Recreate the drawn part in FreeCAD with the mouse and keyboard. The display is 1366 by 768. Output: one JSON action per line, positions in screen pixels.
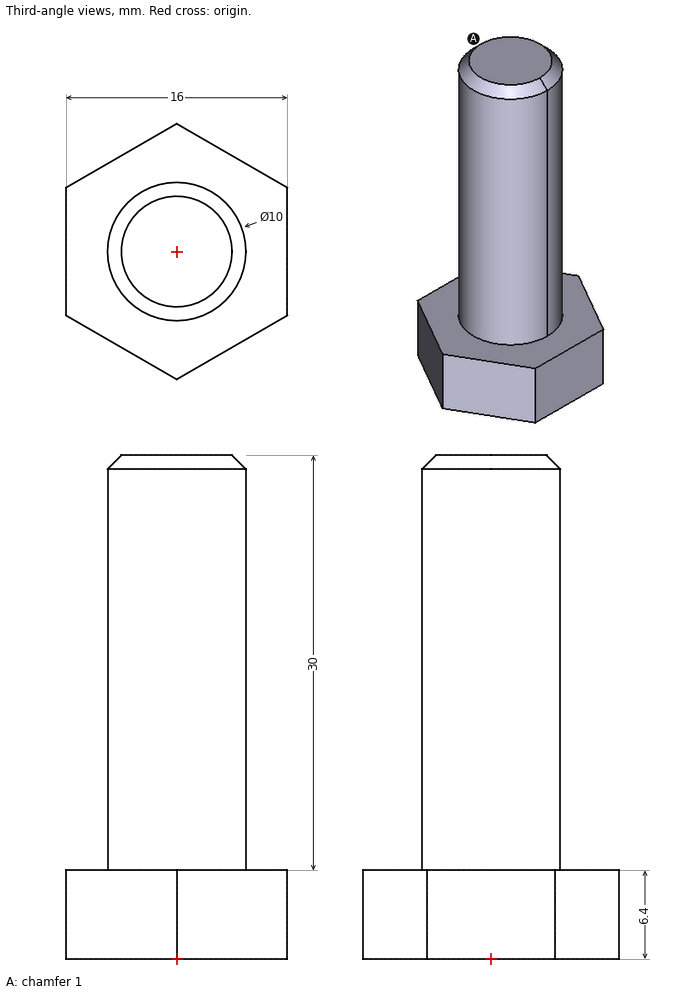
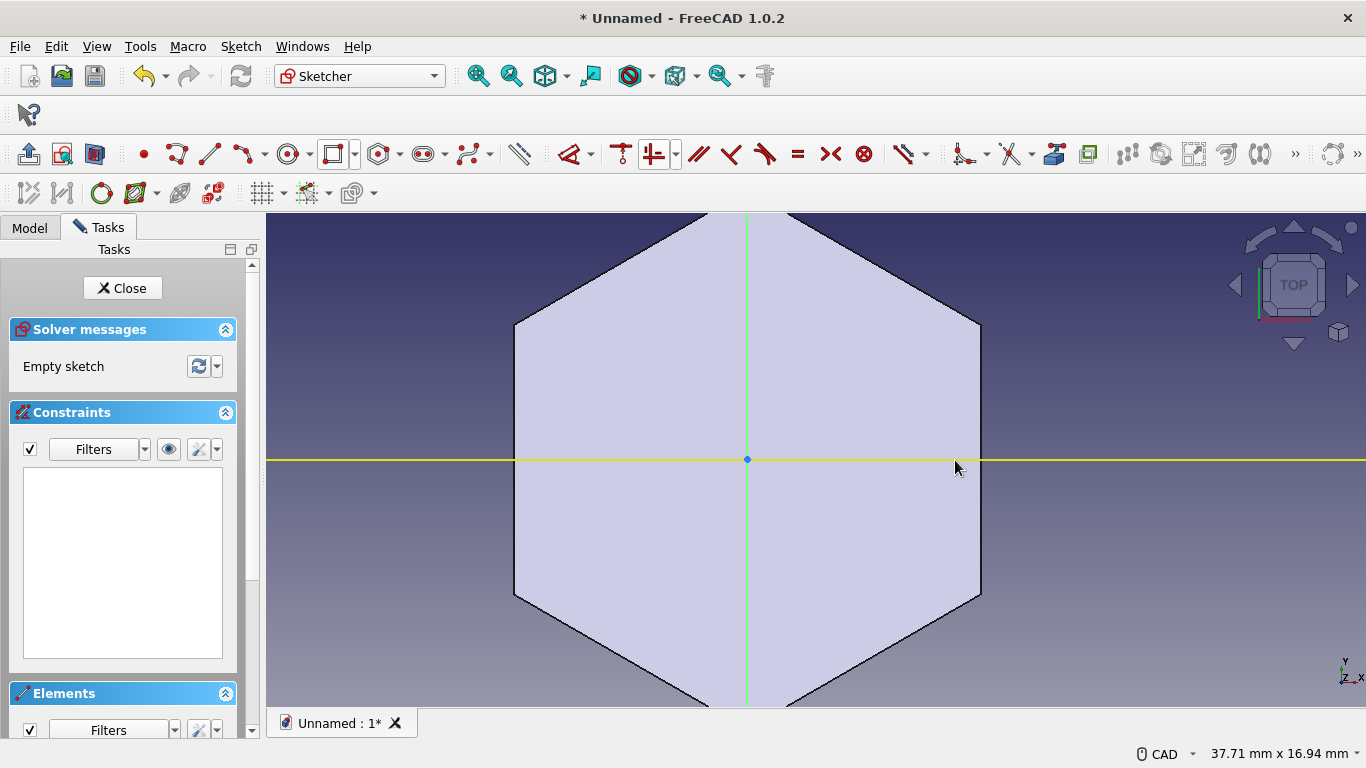
{"action": "key", "text": "g c"}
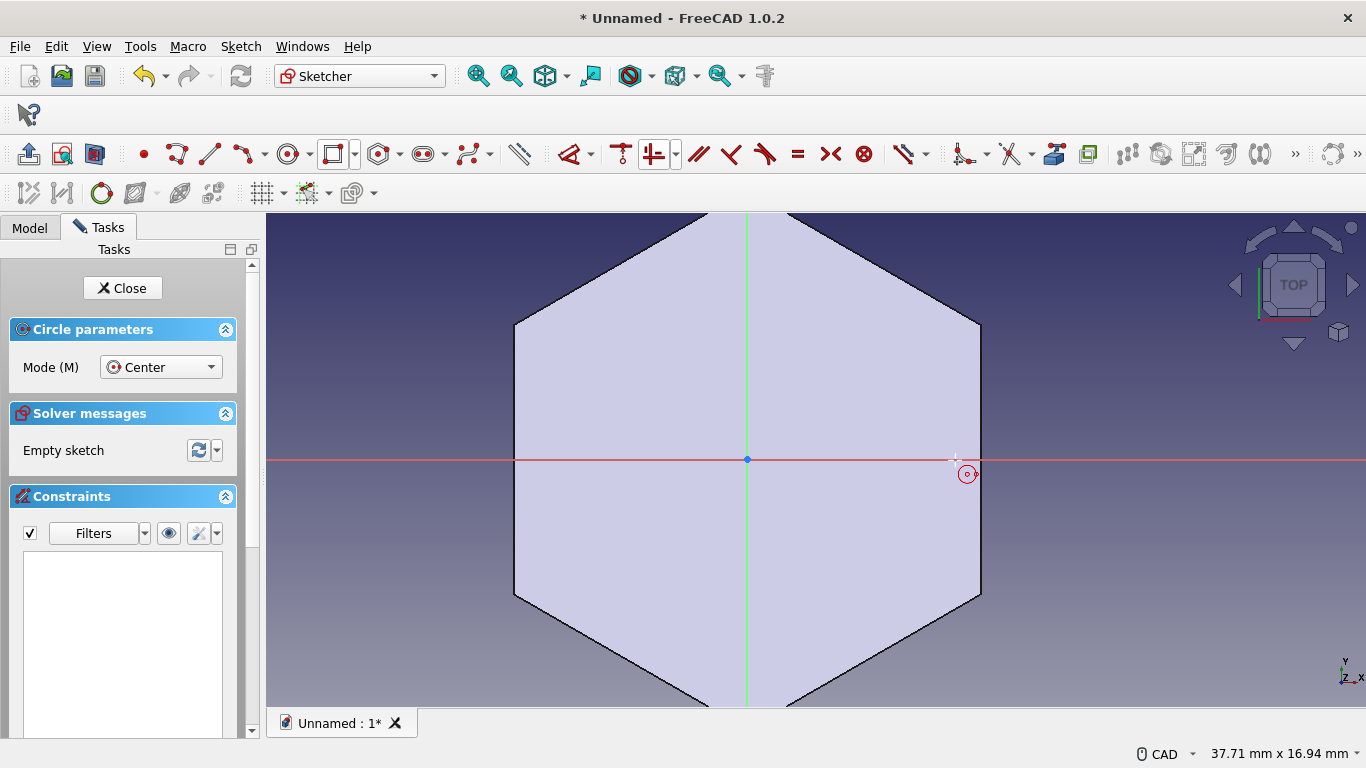
{"action": "left_click", "coordinate": [747, 460]}
{"action": "left_click", "coordinate": [850, 357]}
{"action": "key", "text": "Escape"}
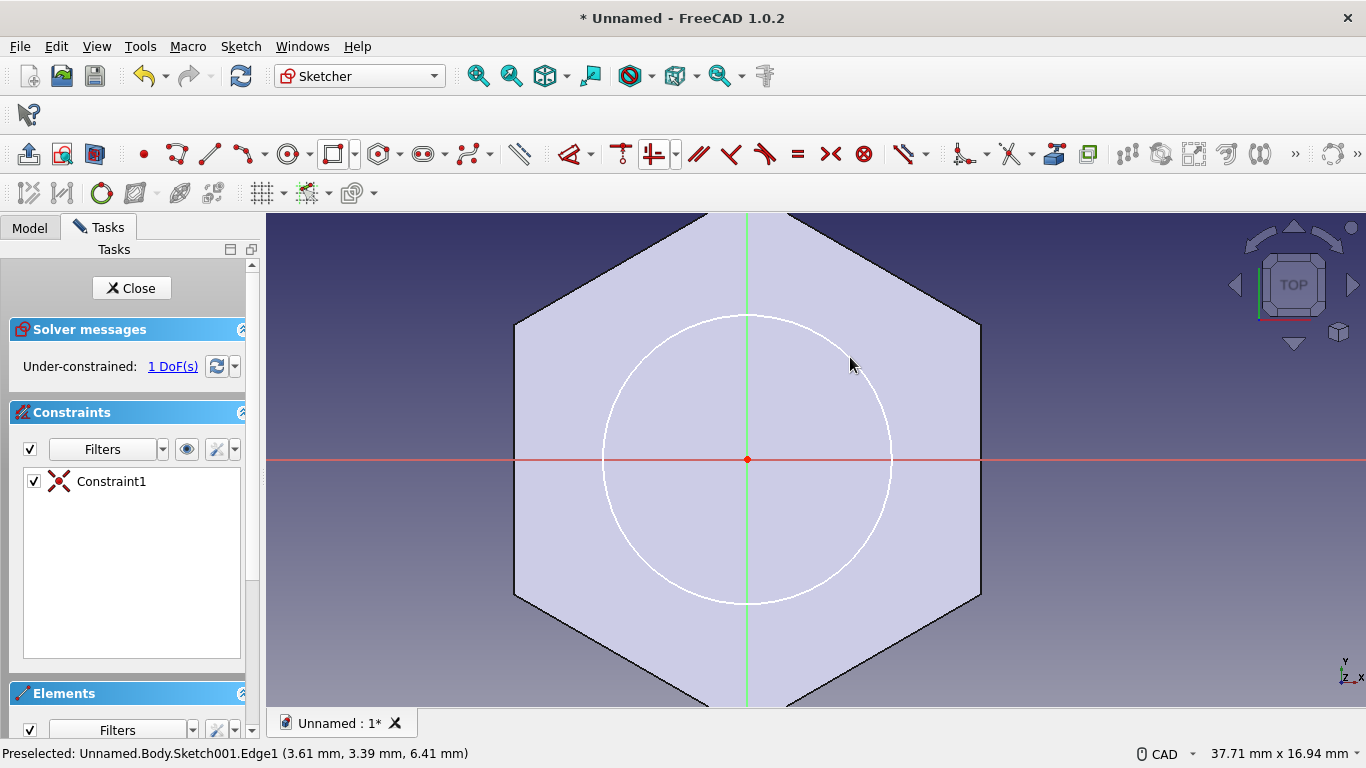
{"action": "key", "text": "d"}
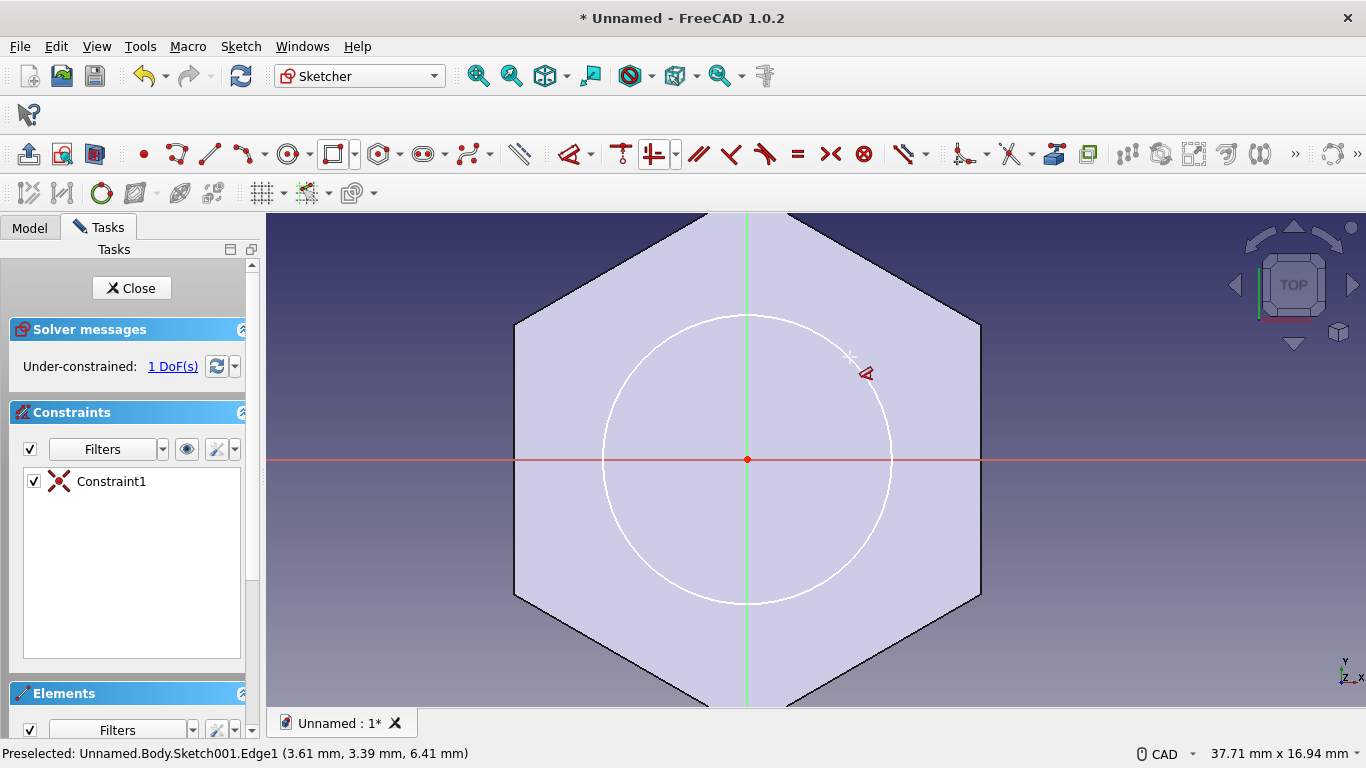
{"action": "left_click", "coordinate": [849, 357]}
{"action": "left_click", "coordinate": [872, 334]}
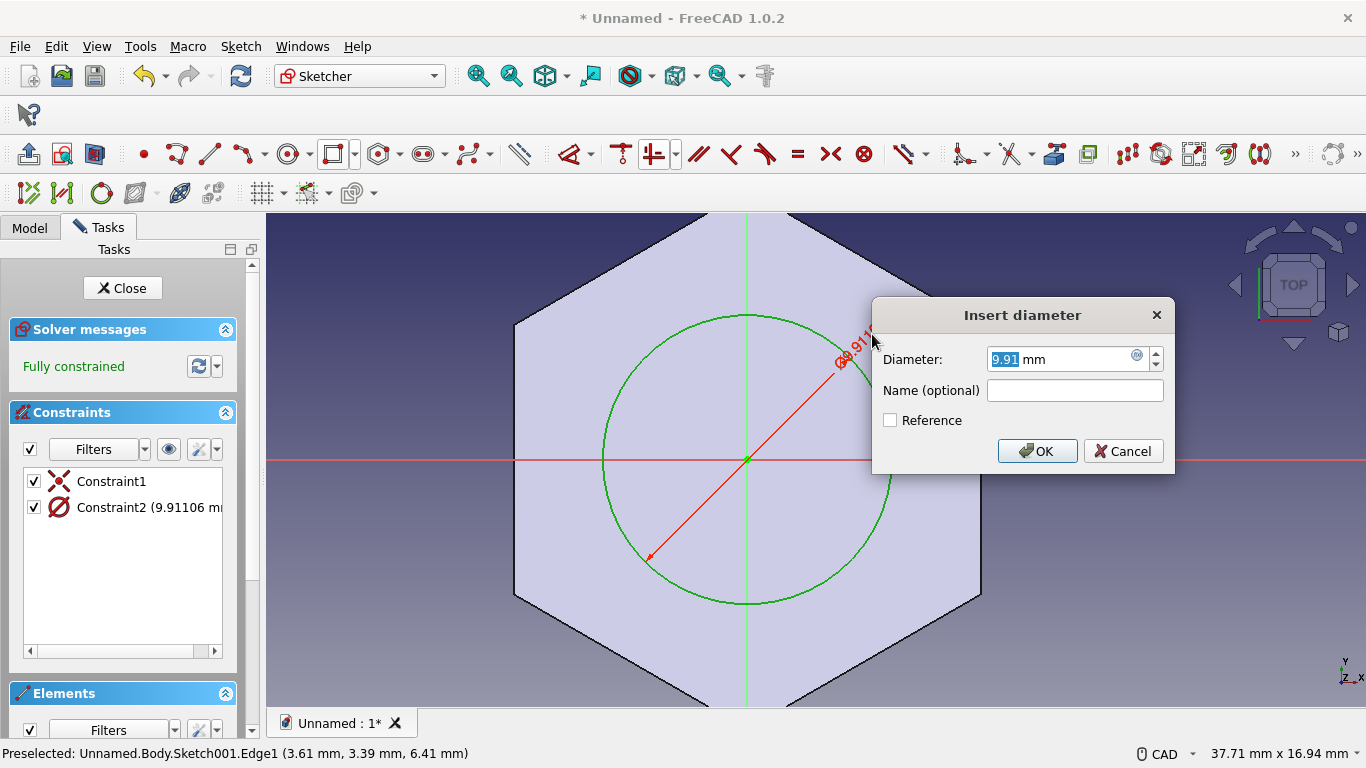
{"action": "type", "text": "10"}
{"action": "key", "text": "Return"}
{"action": "key", "text": "Escape"}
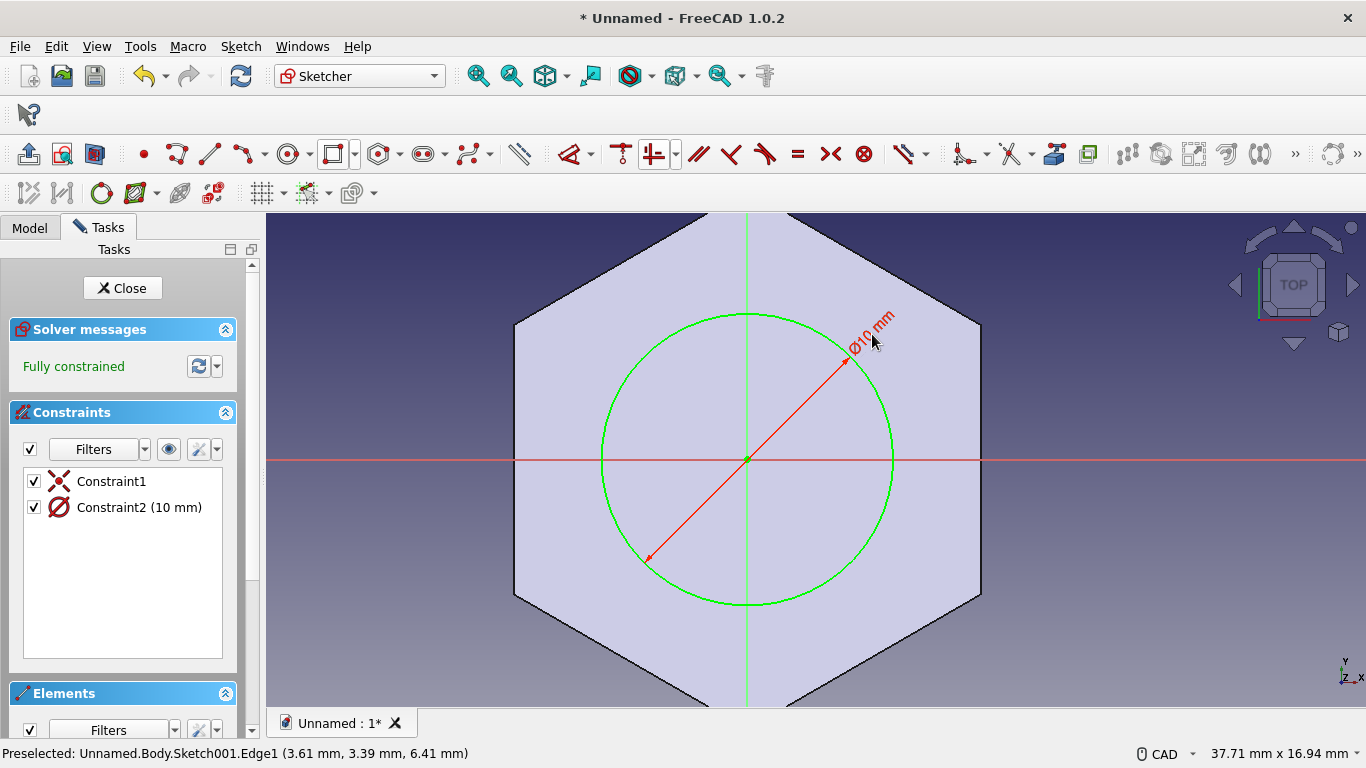
{"action": "left_click", "coordinate": [123, 288]}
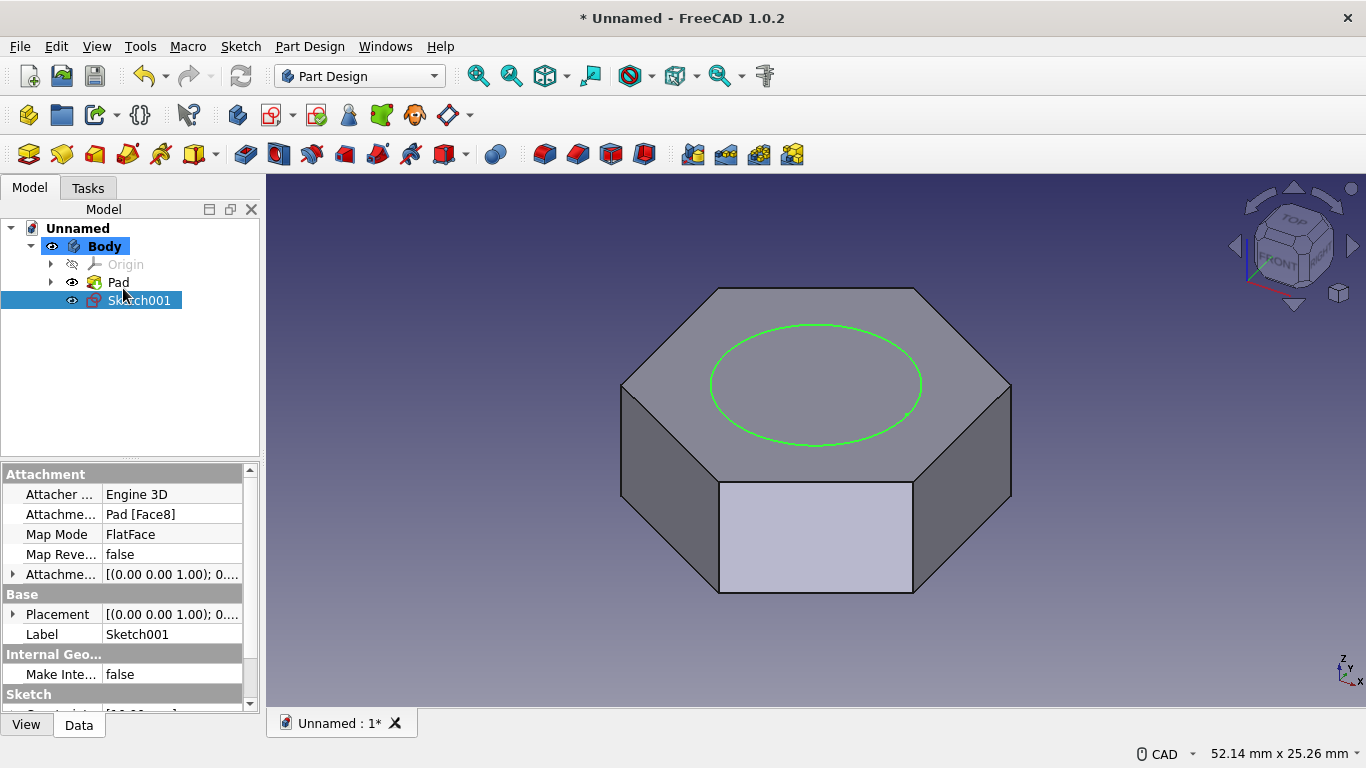
{"action": "left_click", "coordinate": [29, 154]}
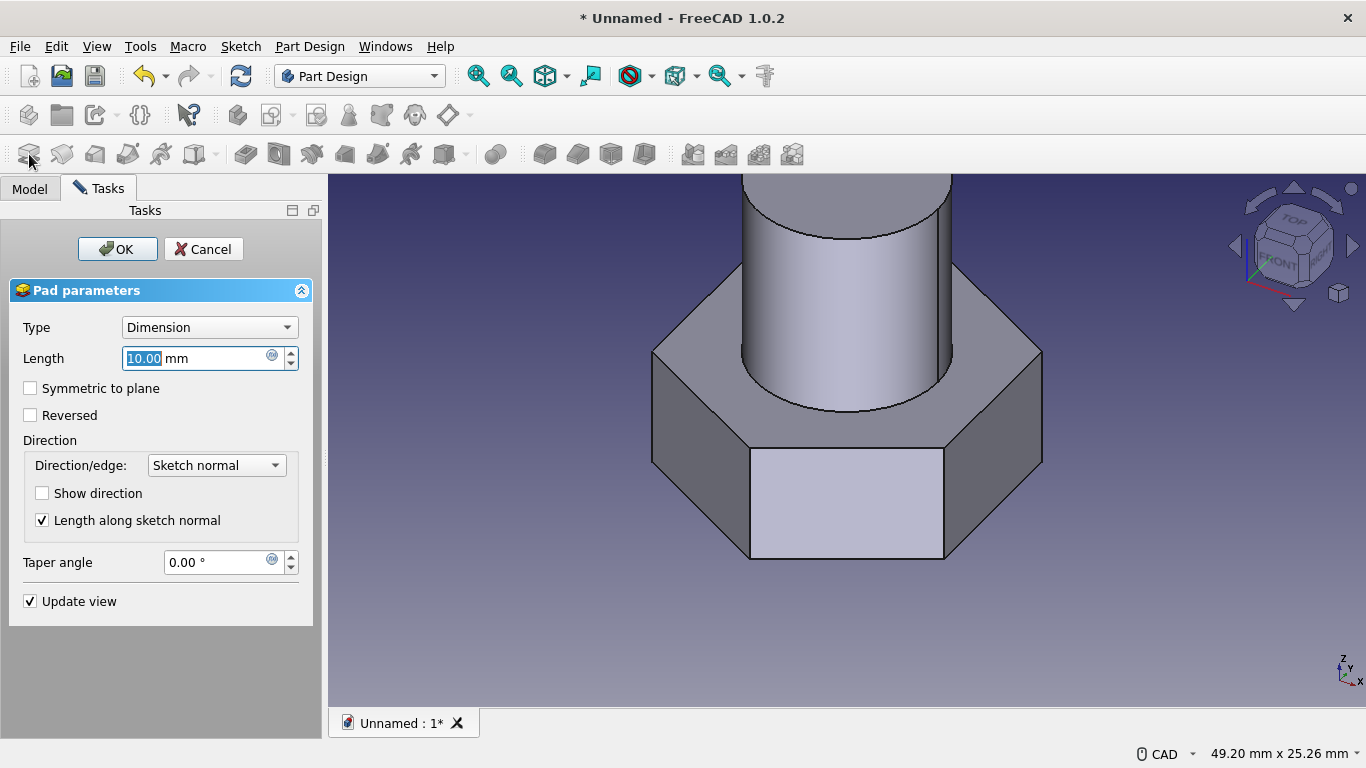
{"action": "type", "text": "30"}
{"action": "key", "text": "Tab"}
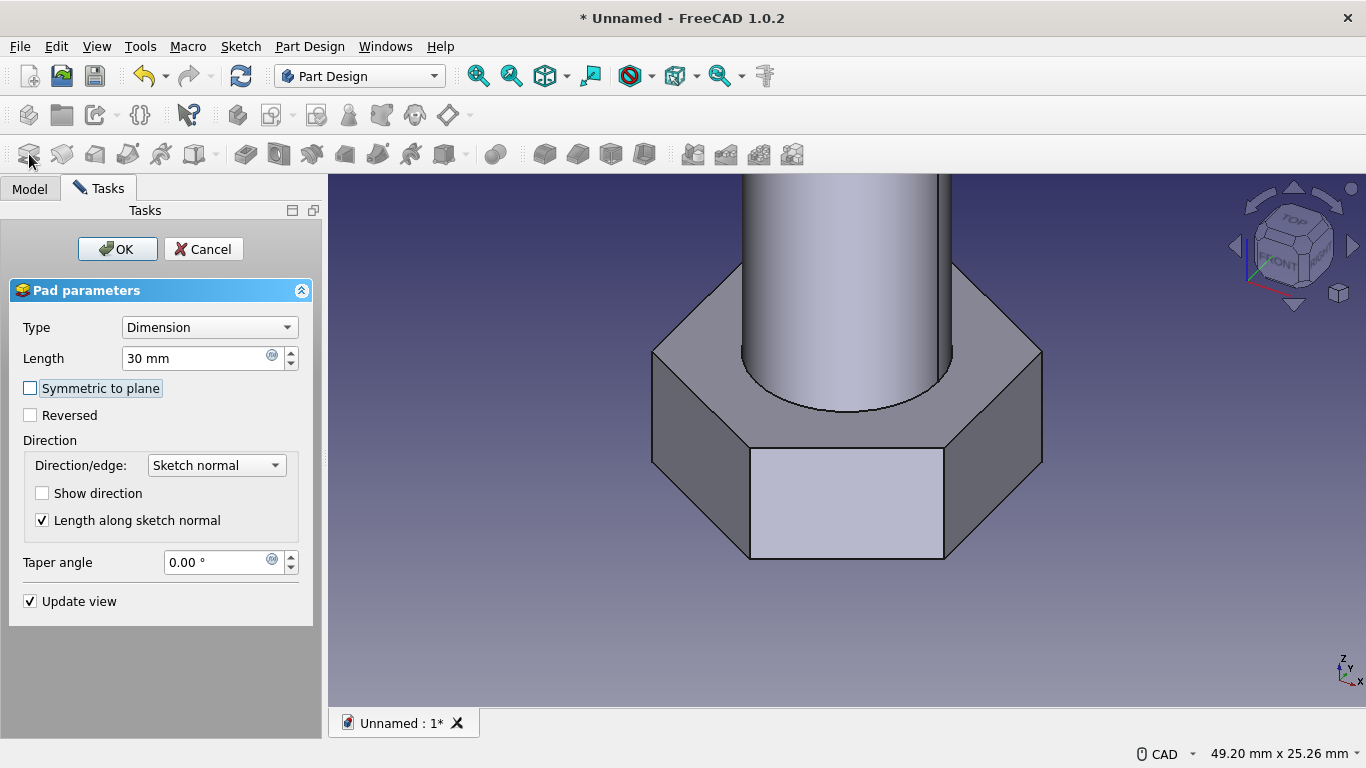
{"action": "left_click", "coordinate": [118, 249]}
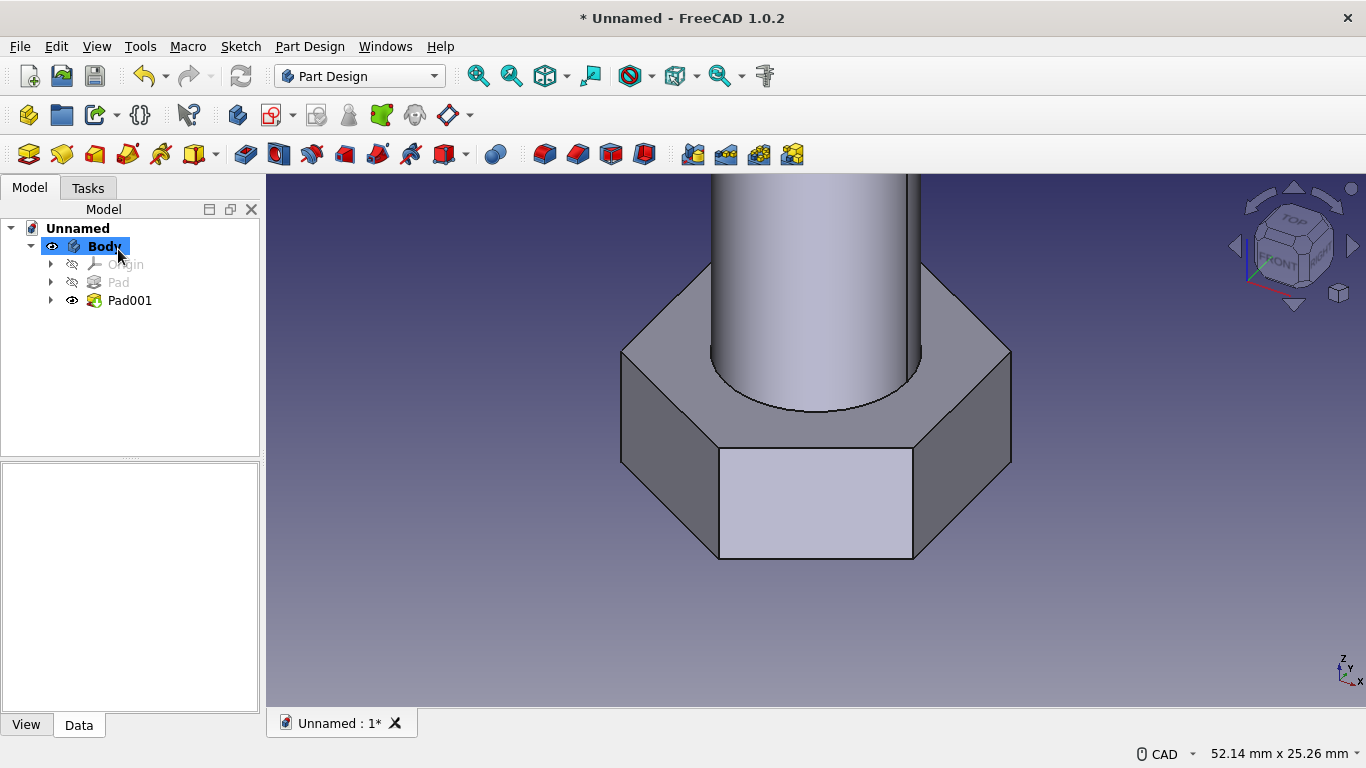
{"action": "key", "text": "v f"}